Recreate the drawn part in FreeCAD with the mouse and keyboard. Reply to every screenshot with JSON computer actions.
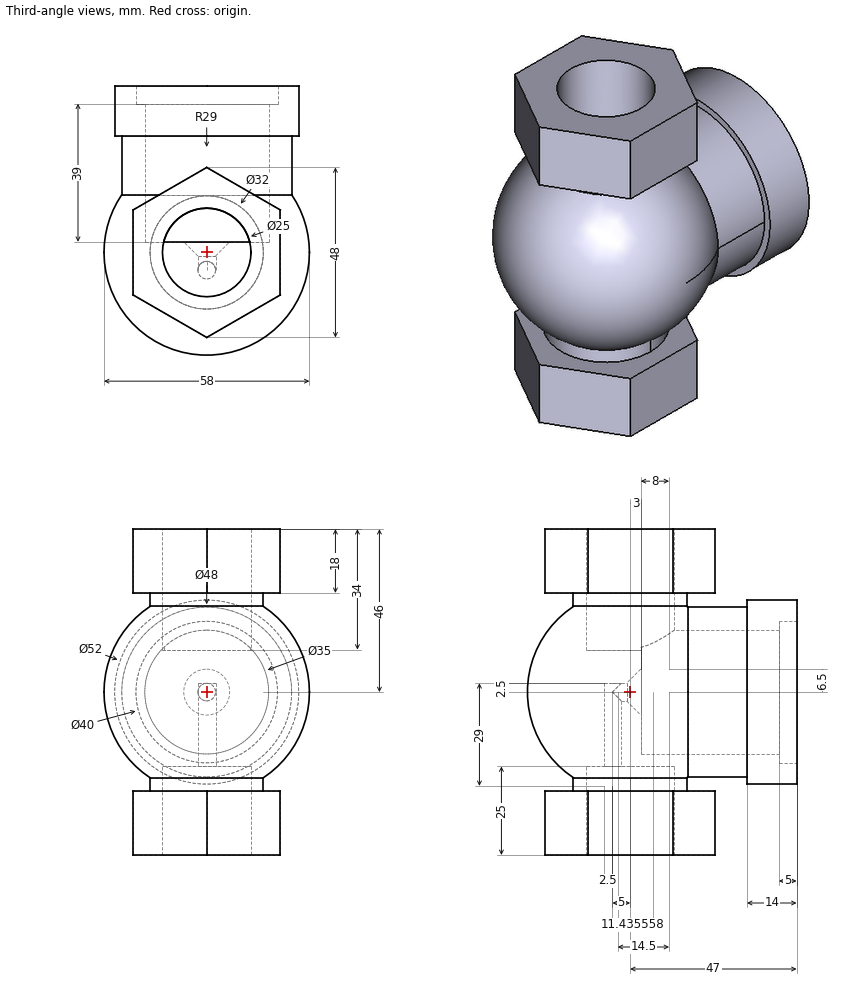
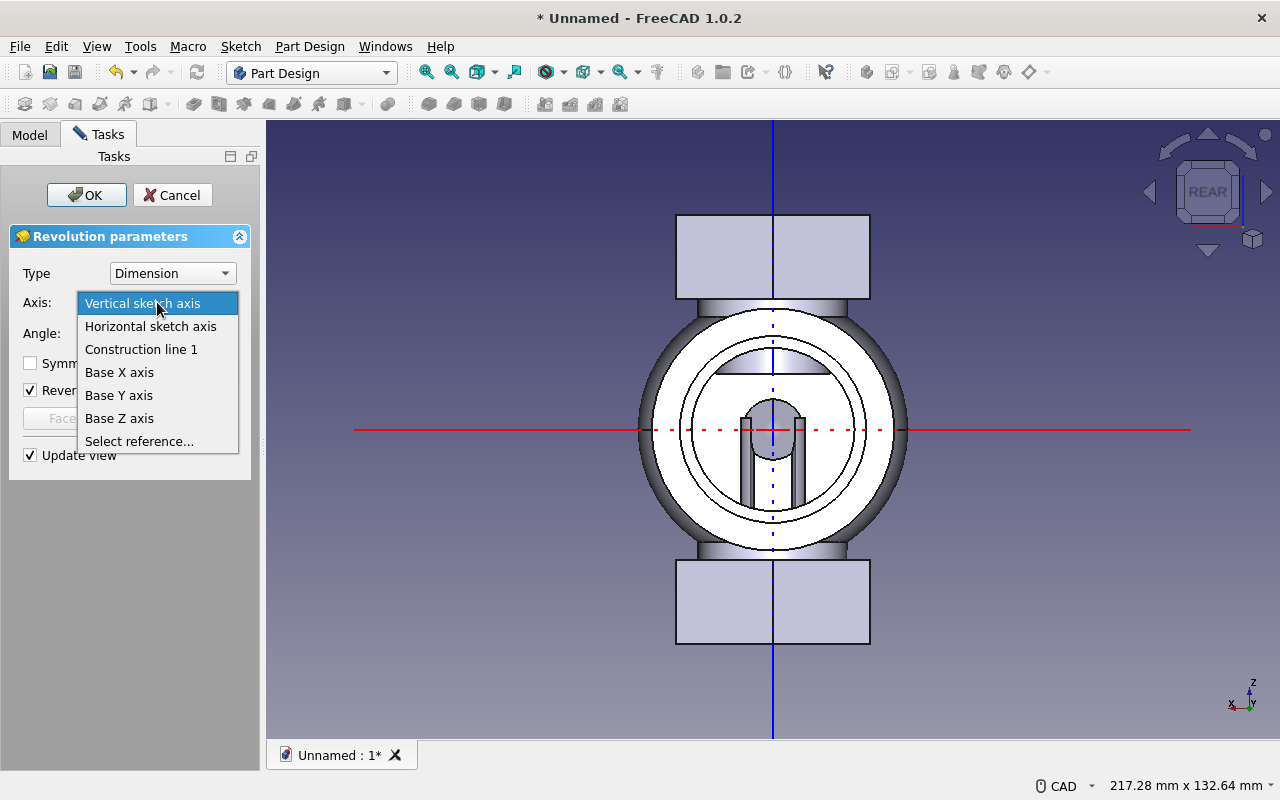
{"action": "left_click", "coordinate": [156, 350]}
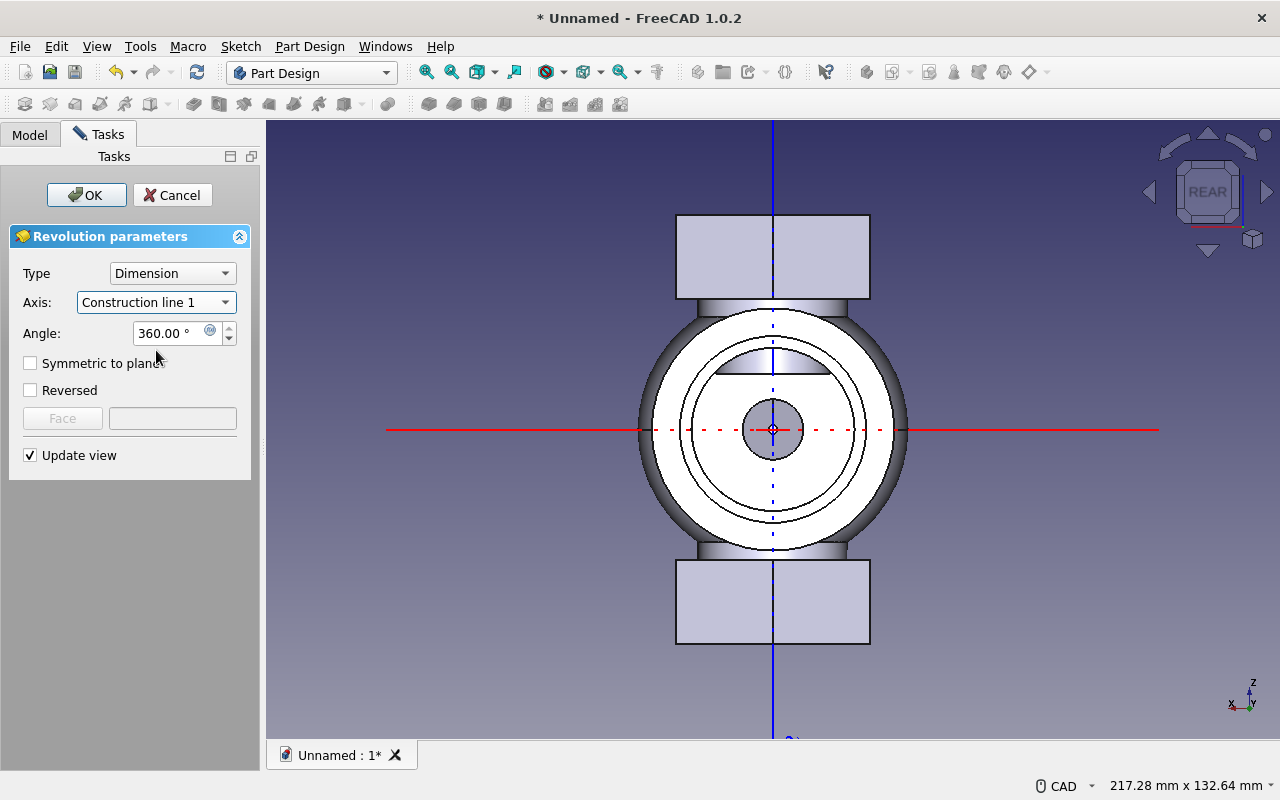
{"action": "left_click", "coordinate": [87, 195]}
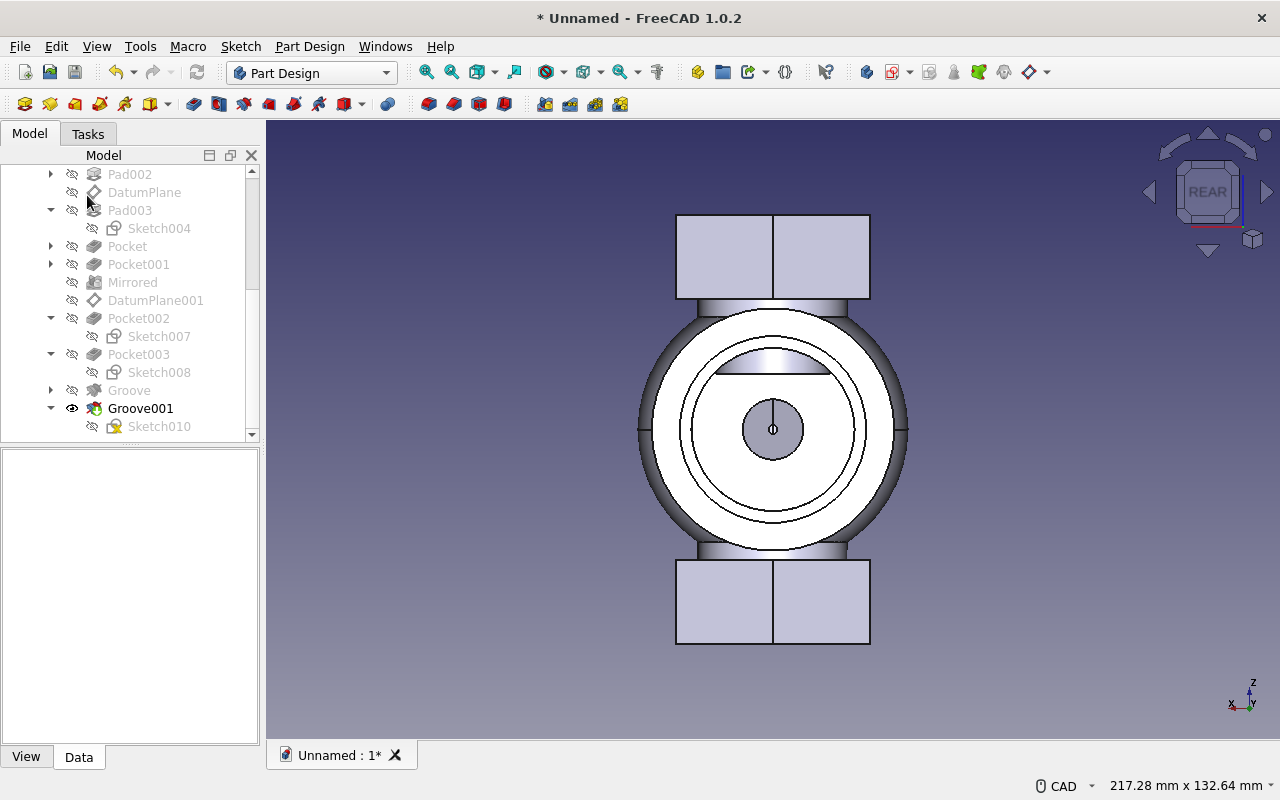
{"action": "left_click", "coordinate": [892, 72]}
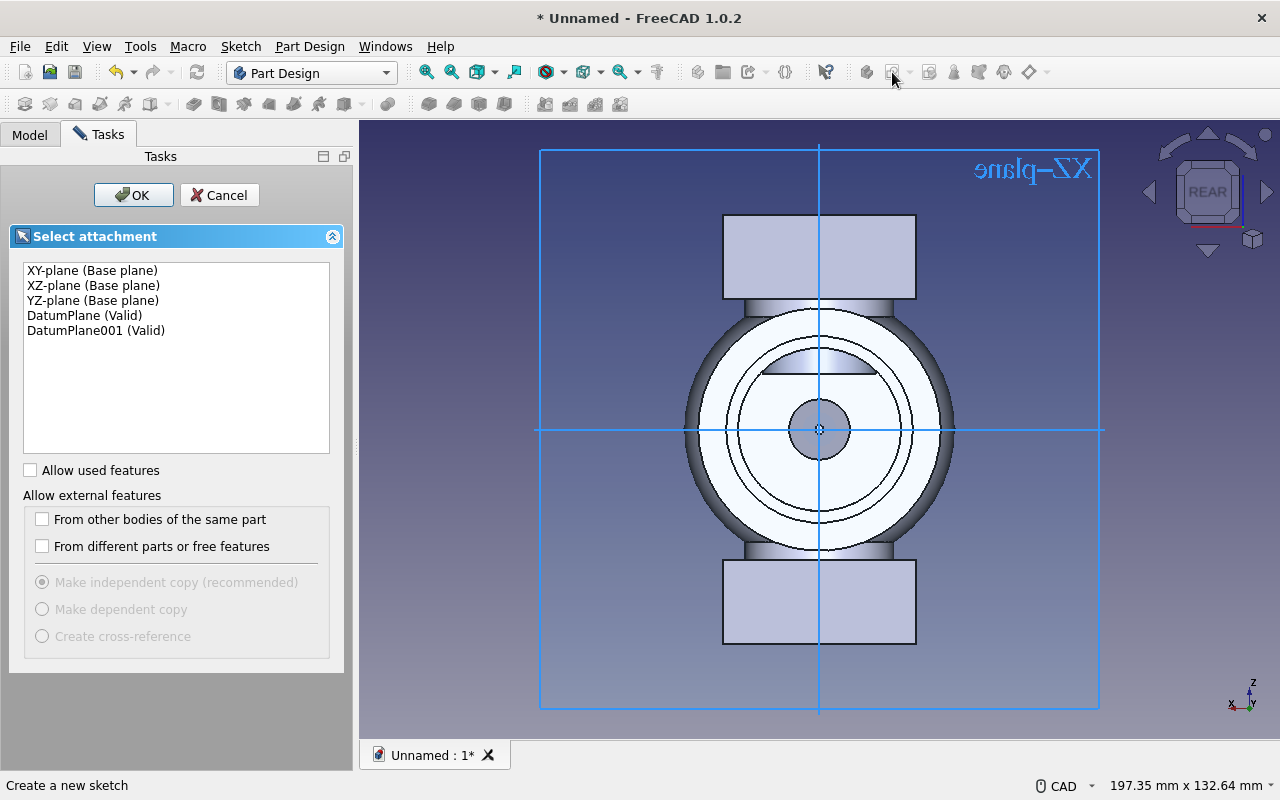
{"action": "left_click", "coordinate": [84, 300]}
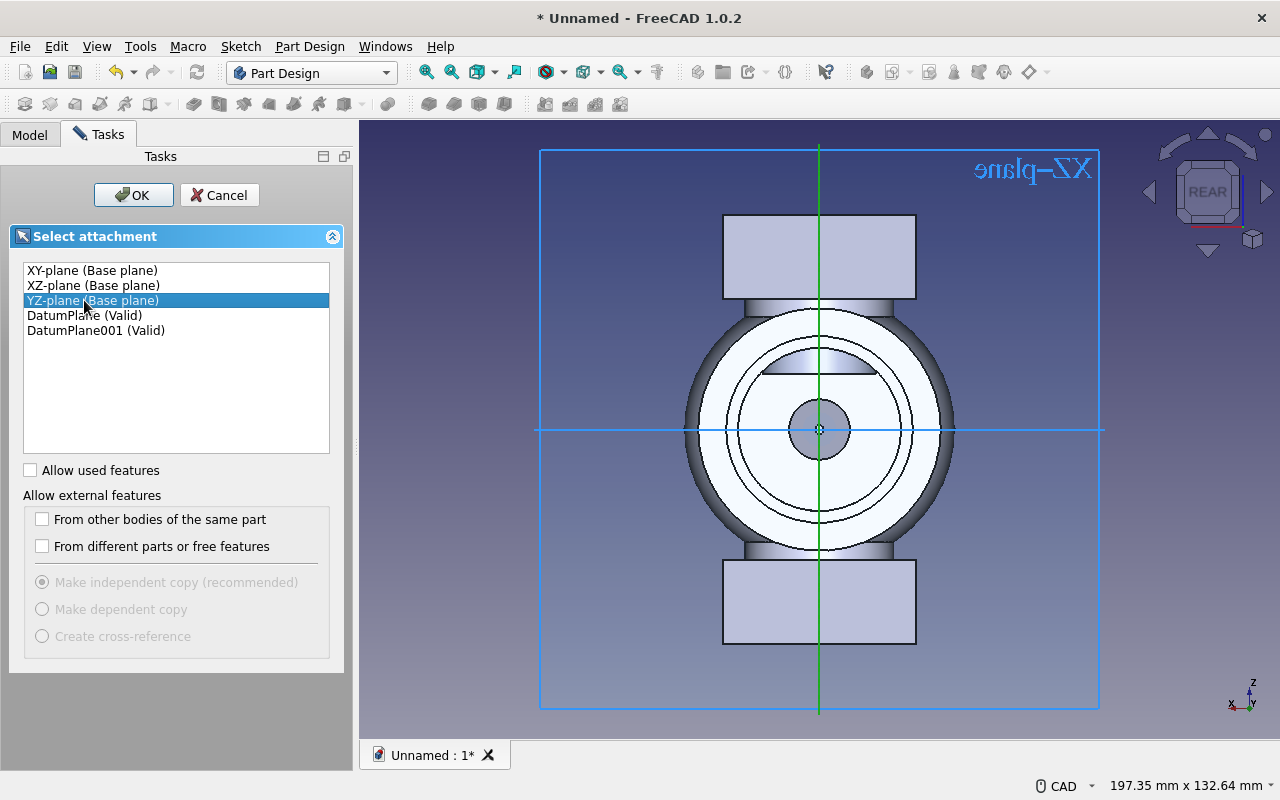
{"action": "left_click", "coordinate": [134, 195]}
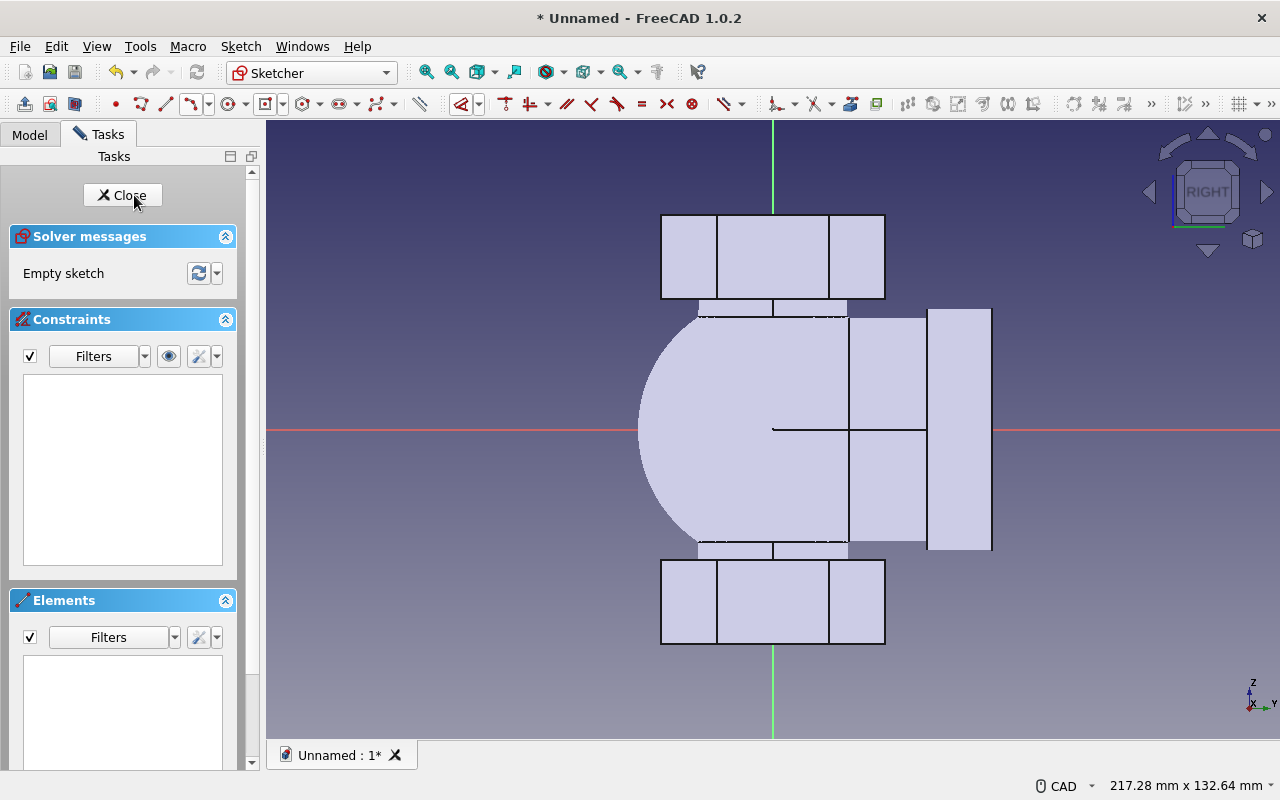
{"action": "left_click", "coordinate": [75, 104]}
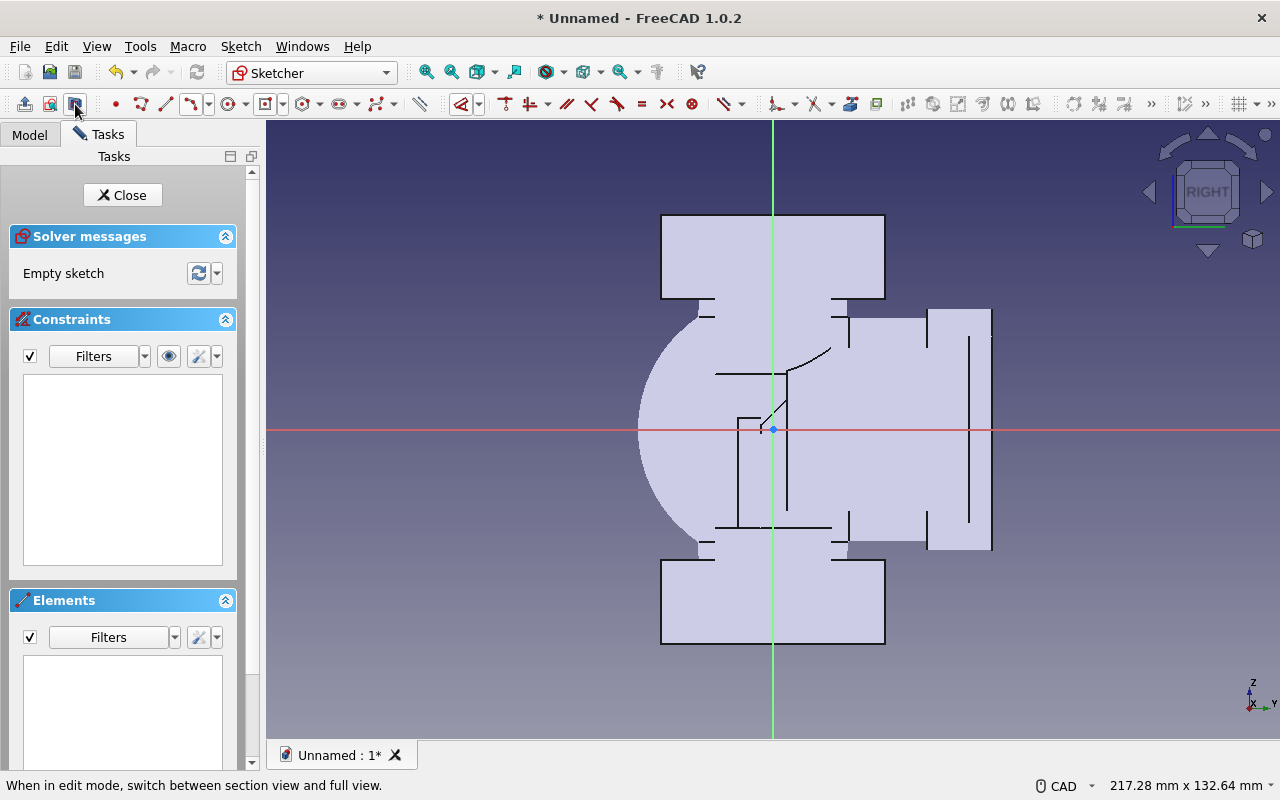
{"action": "scroll", "coordinate": [784, 423], "scroll_direction": "up", "scroll_amount": 12}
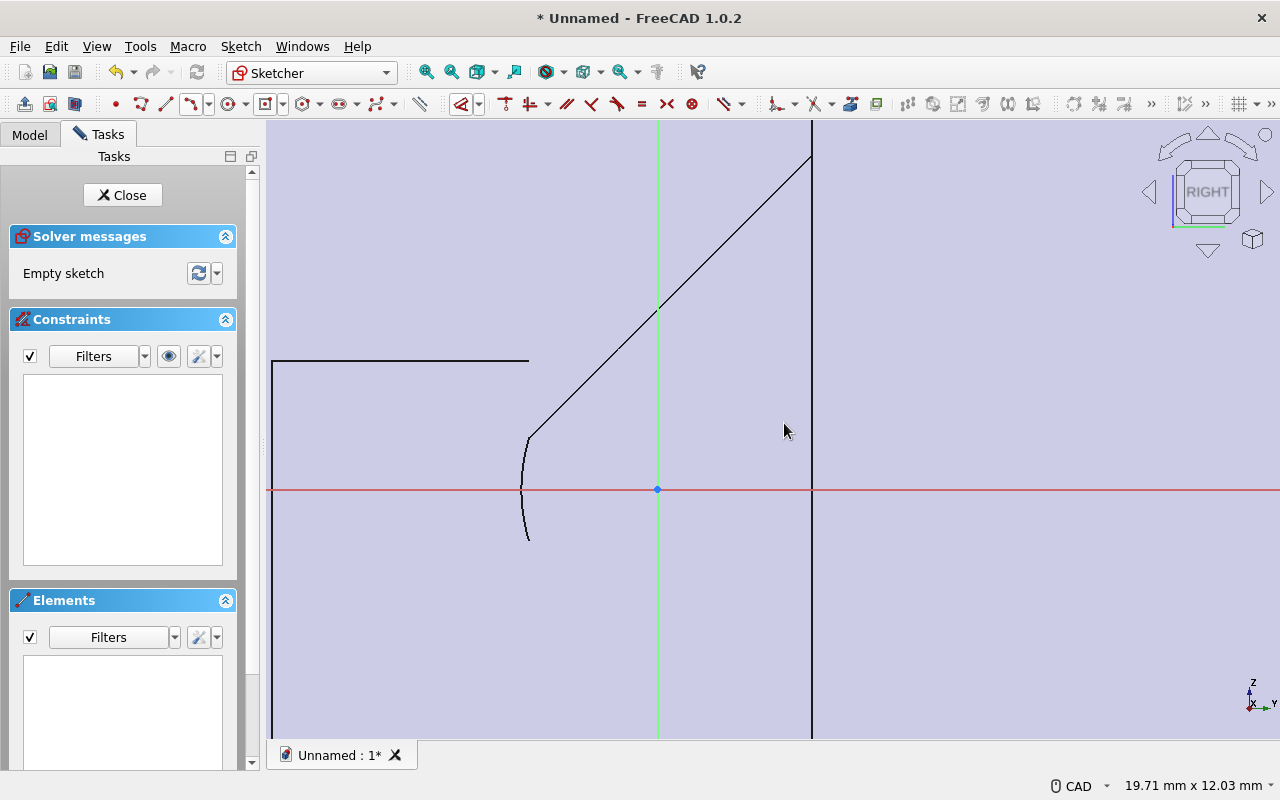
{"action": "key", "text": "g r"}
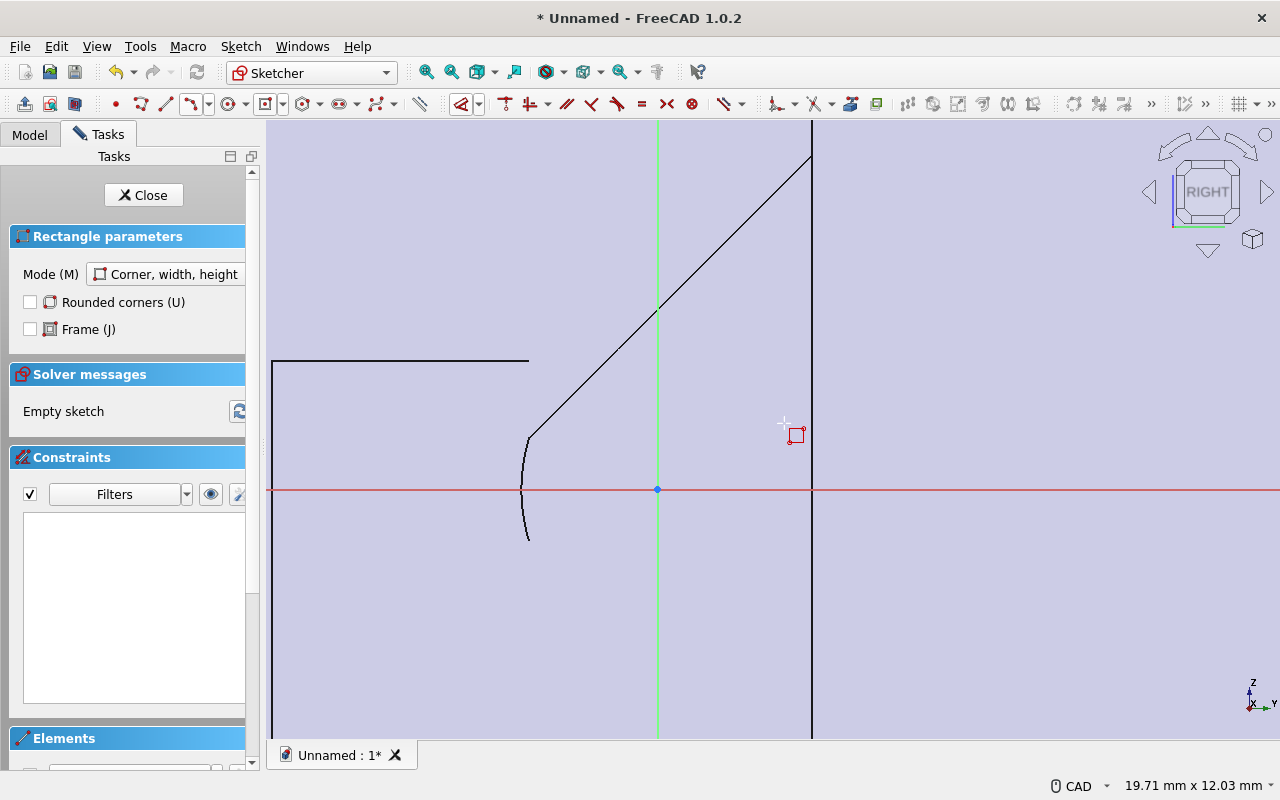
{"action": "left_click", "coordinate": [400, 361]}
{"action": "left_click", "coordinate": [989, 490]}
{"action": "key", "text": "Escape"}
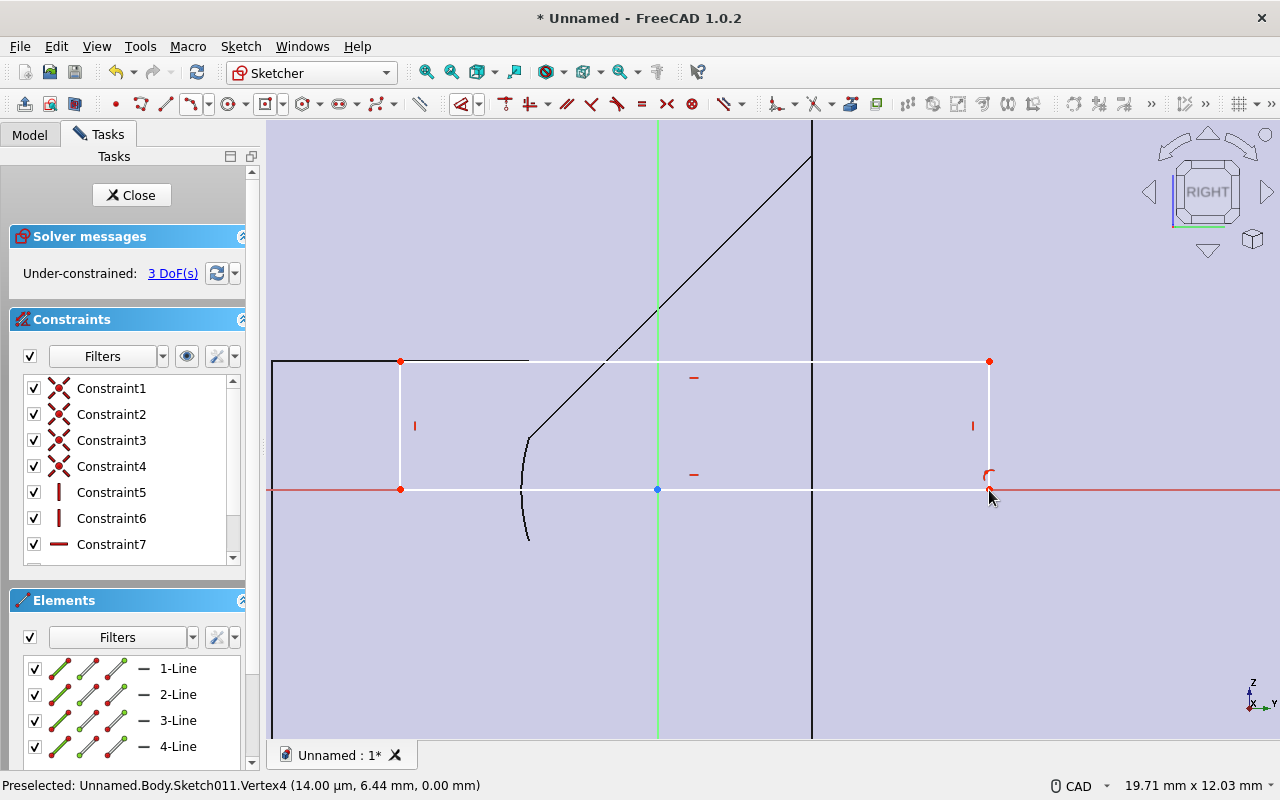
{"action": "left_click", "coordinate": [400, 362]}